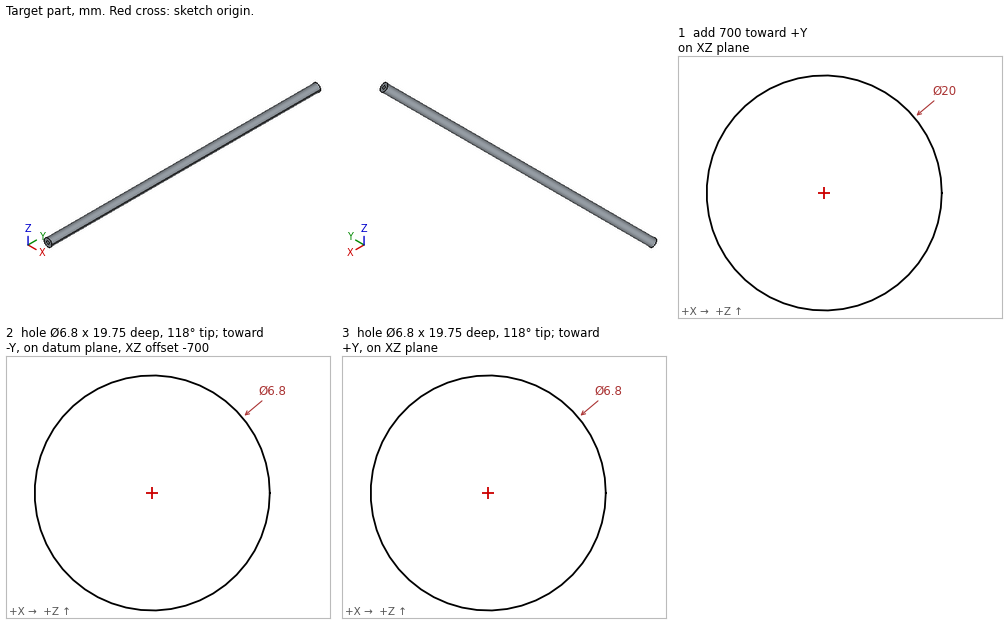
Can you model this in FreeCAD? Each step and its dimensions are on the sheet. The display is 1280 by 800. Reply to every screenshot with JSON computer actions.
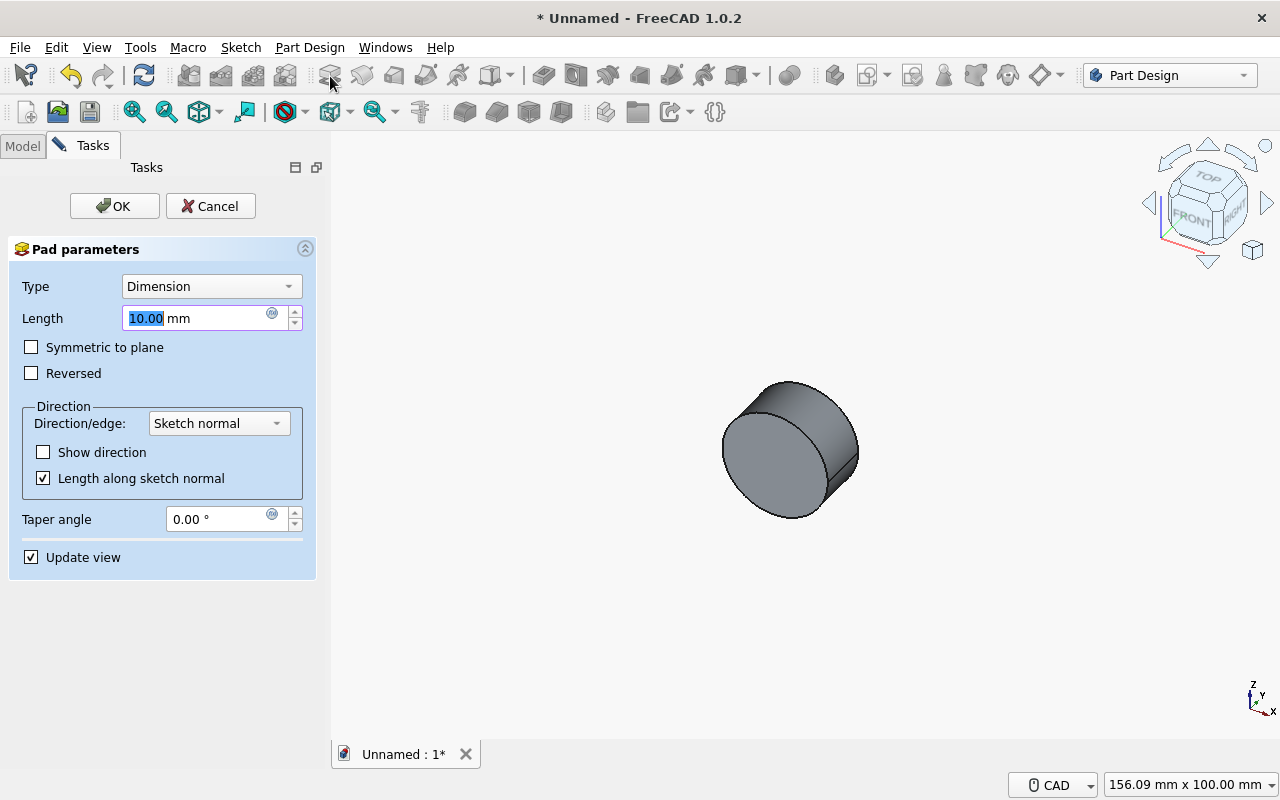
{"action": "type", "text": "700"}
{"action": "key", "text": "Tab"}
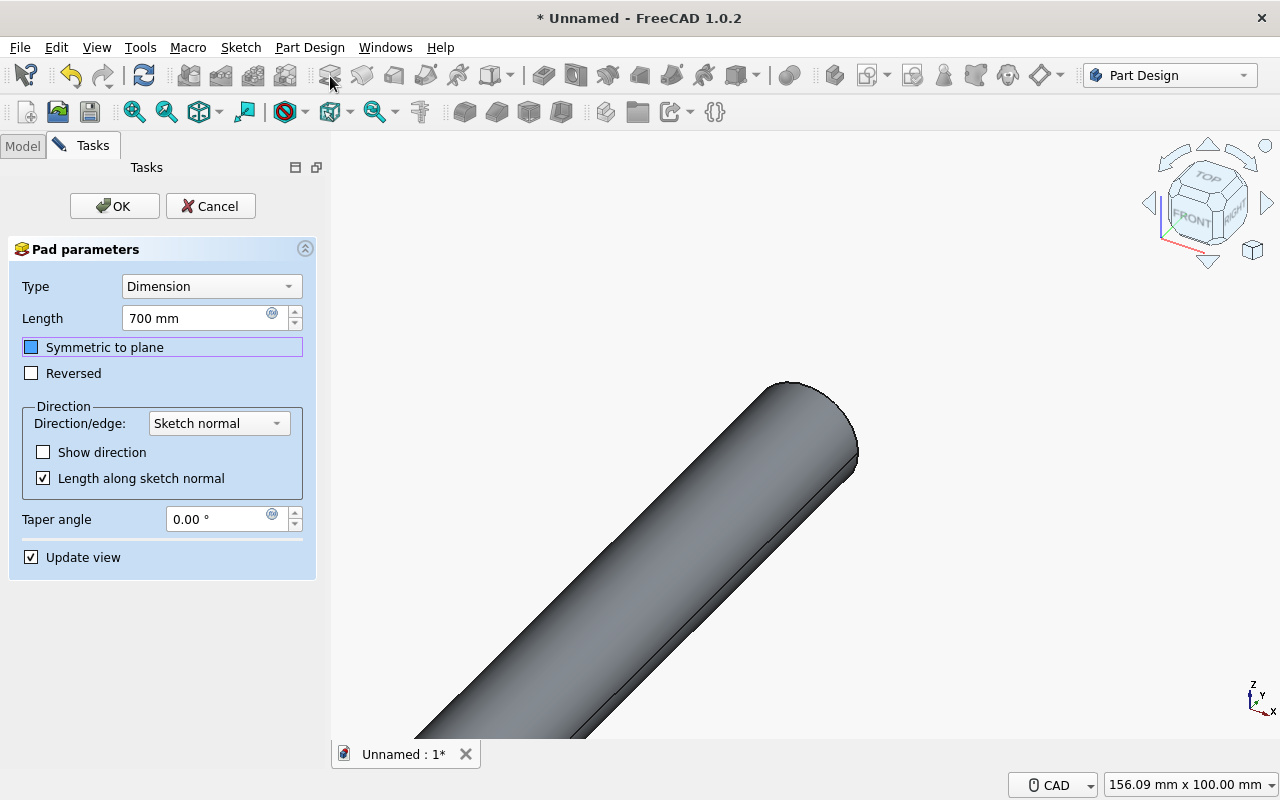
{"action": "left_click", "coordinate": [30, 373]}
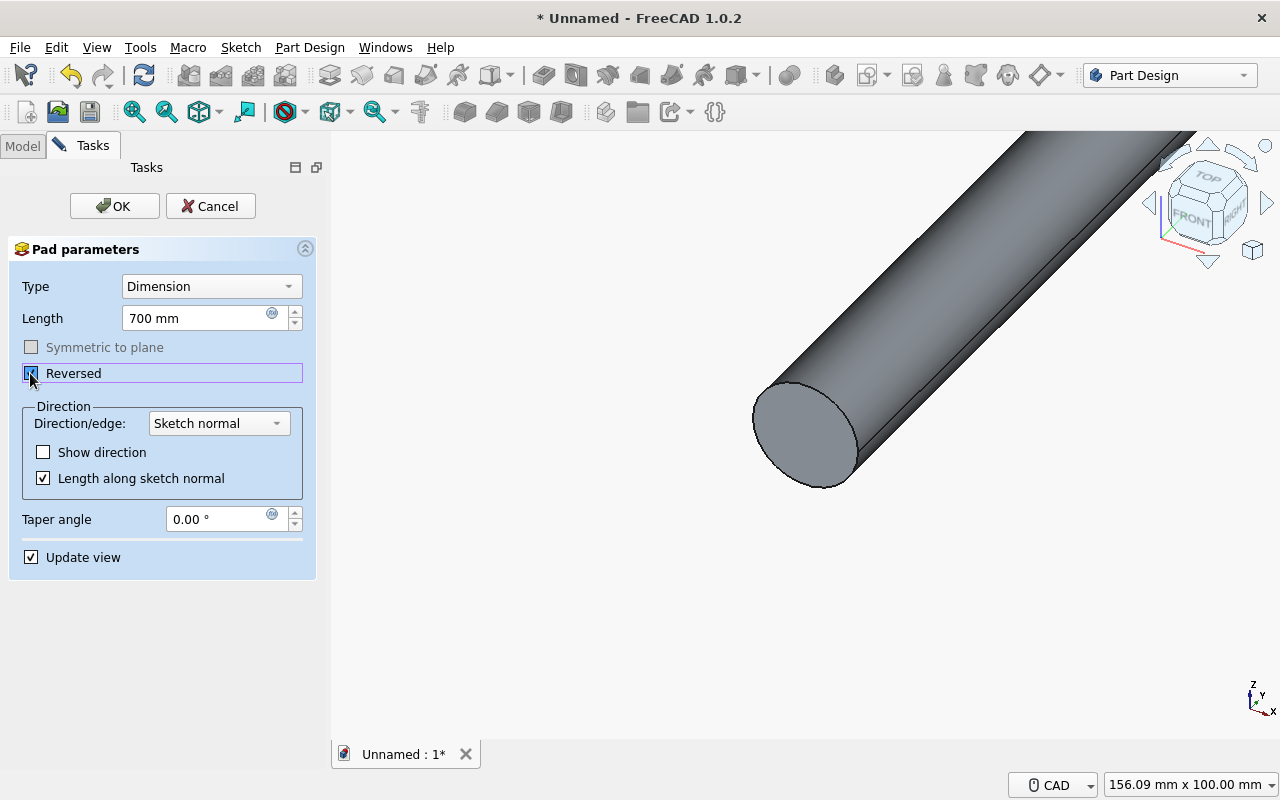
{"action": "left_click", "coordinate": [115, 206]}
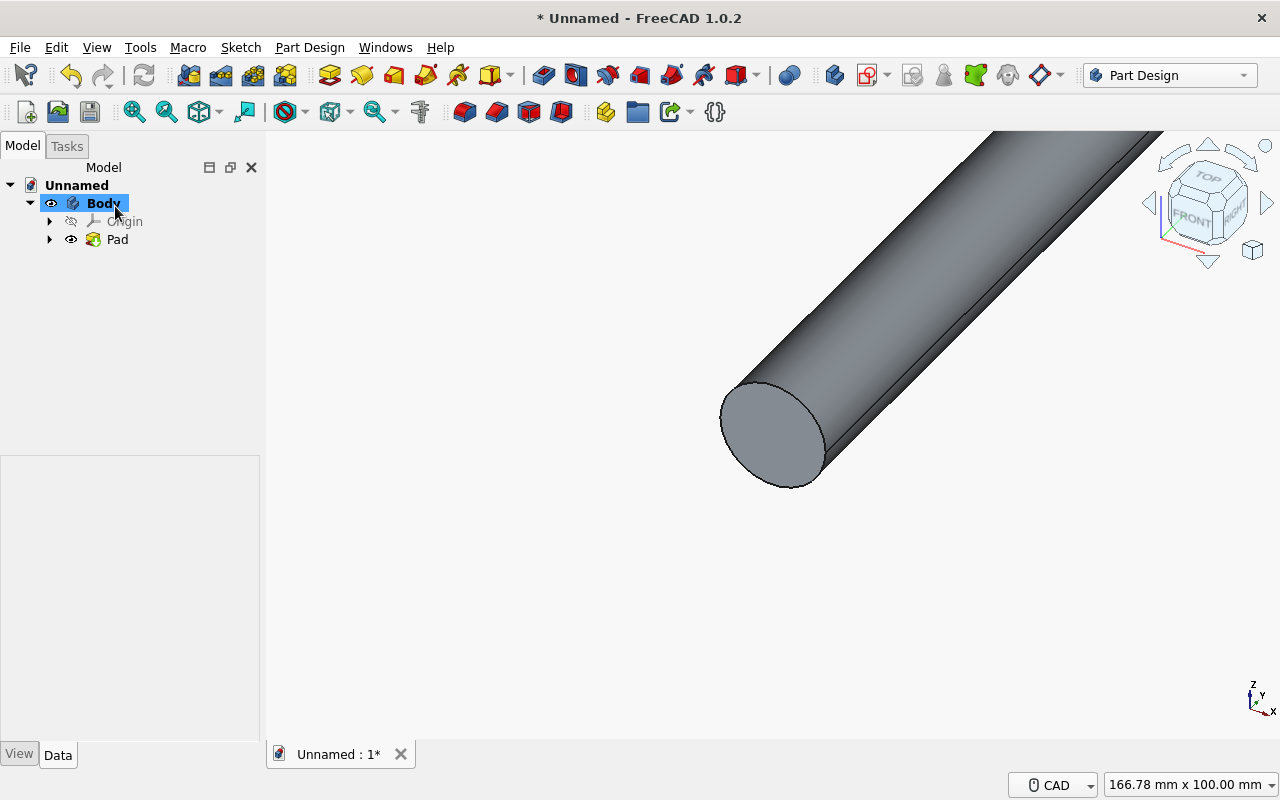
{"action": "left_click", "coordinate": [136, 112]}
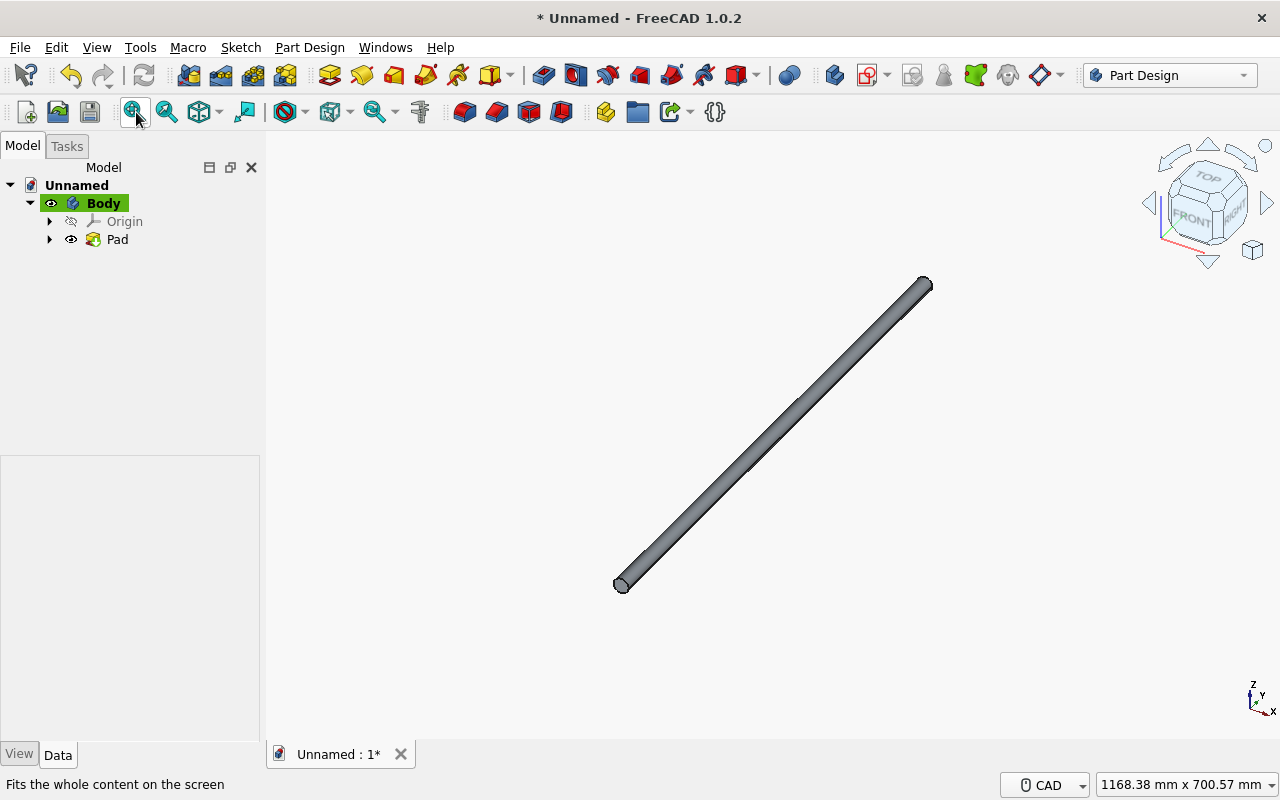
{"action": "key", "text": "4"}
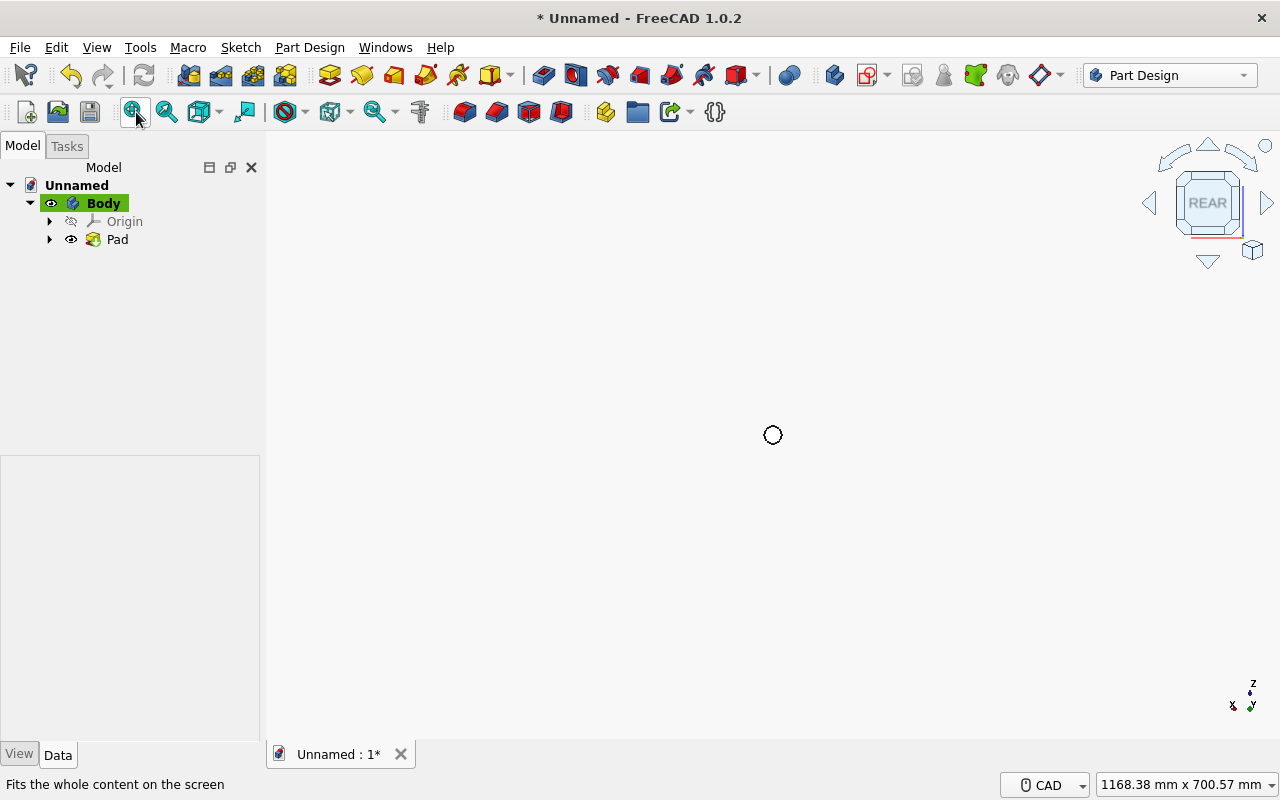
{"action": "left_click", "coordinate": [136, 112]}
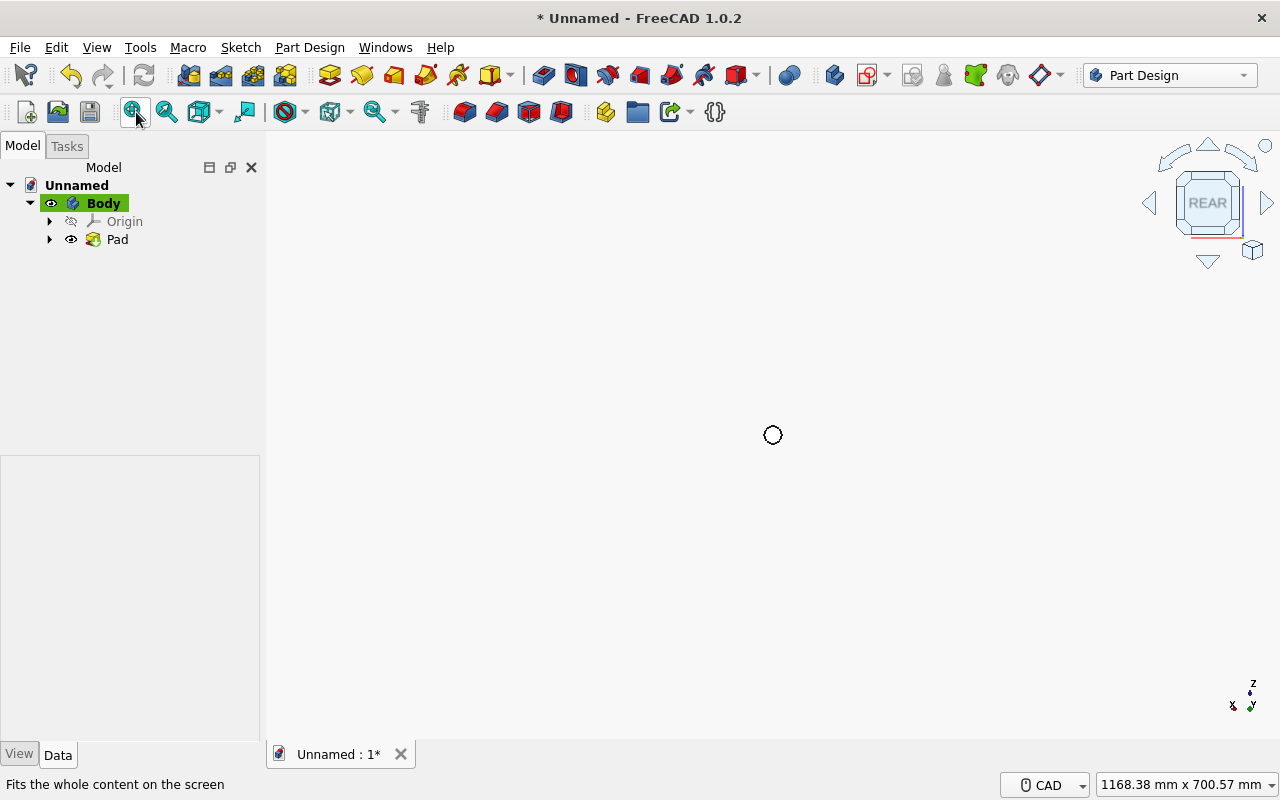
{"action": "key", "text": "5"}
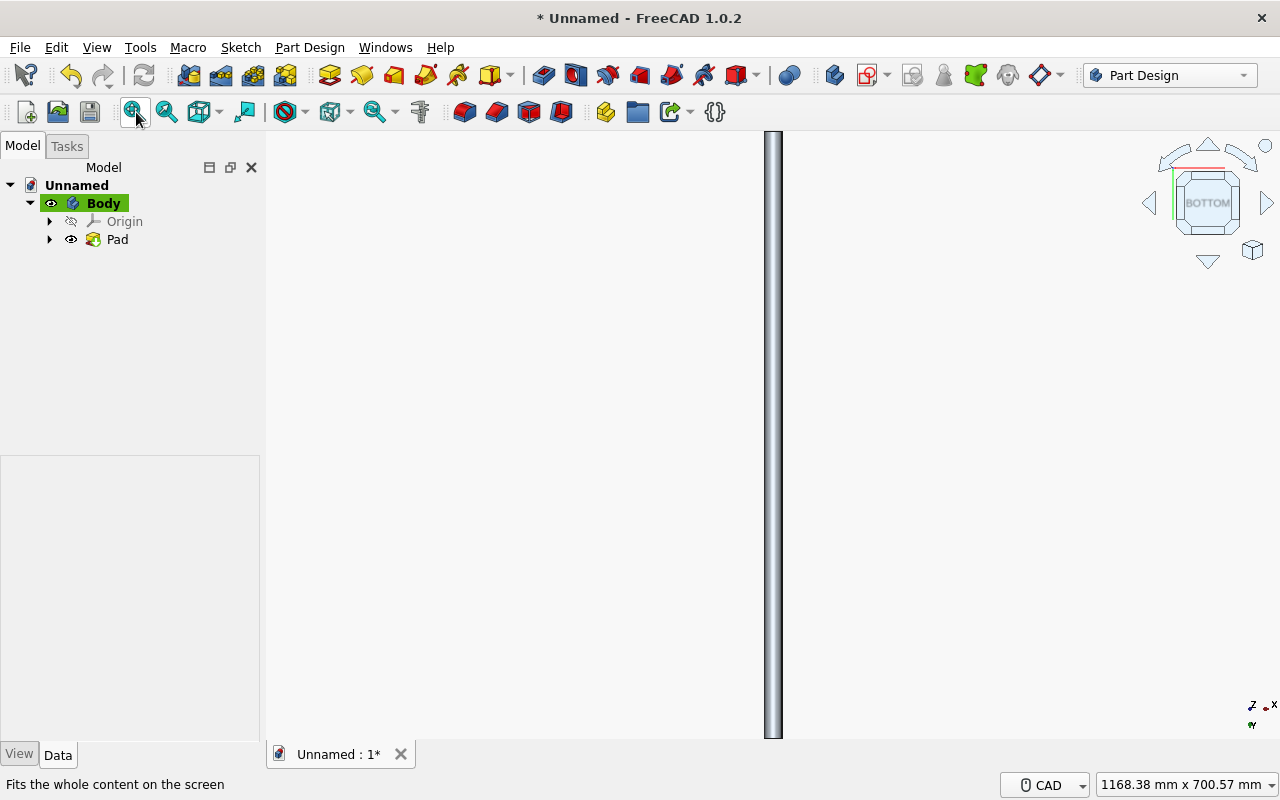
{"action": "left_click", "coordinate": [136, 112]}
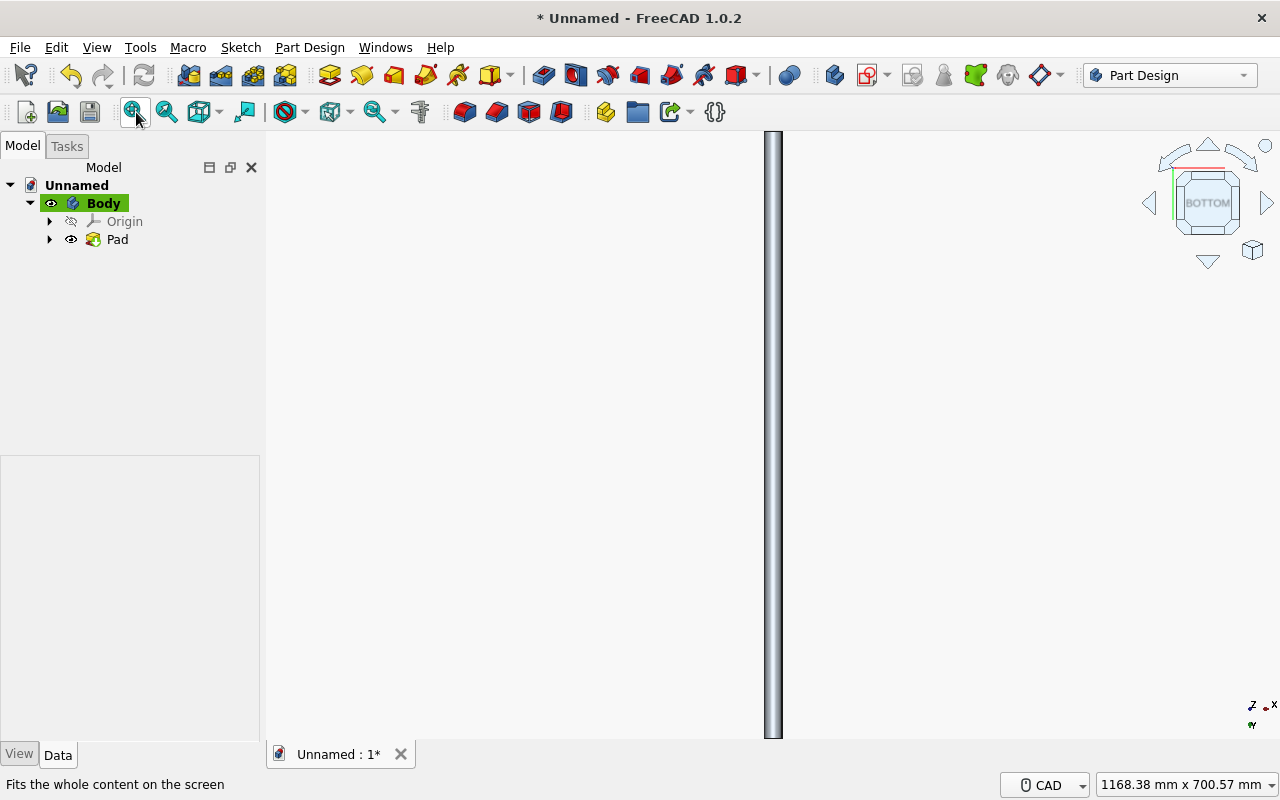
{"action": "key", "text": "3"}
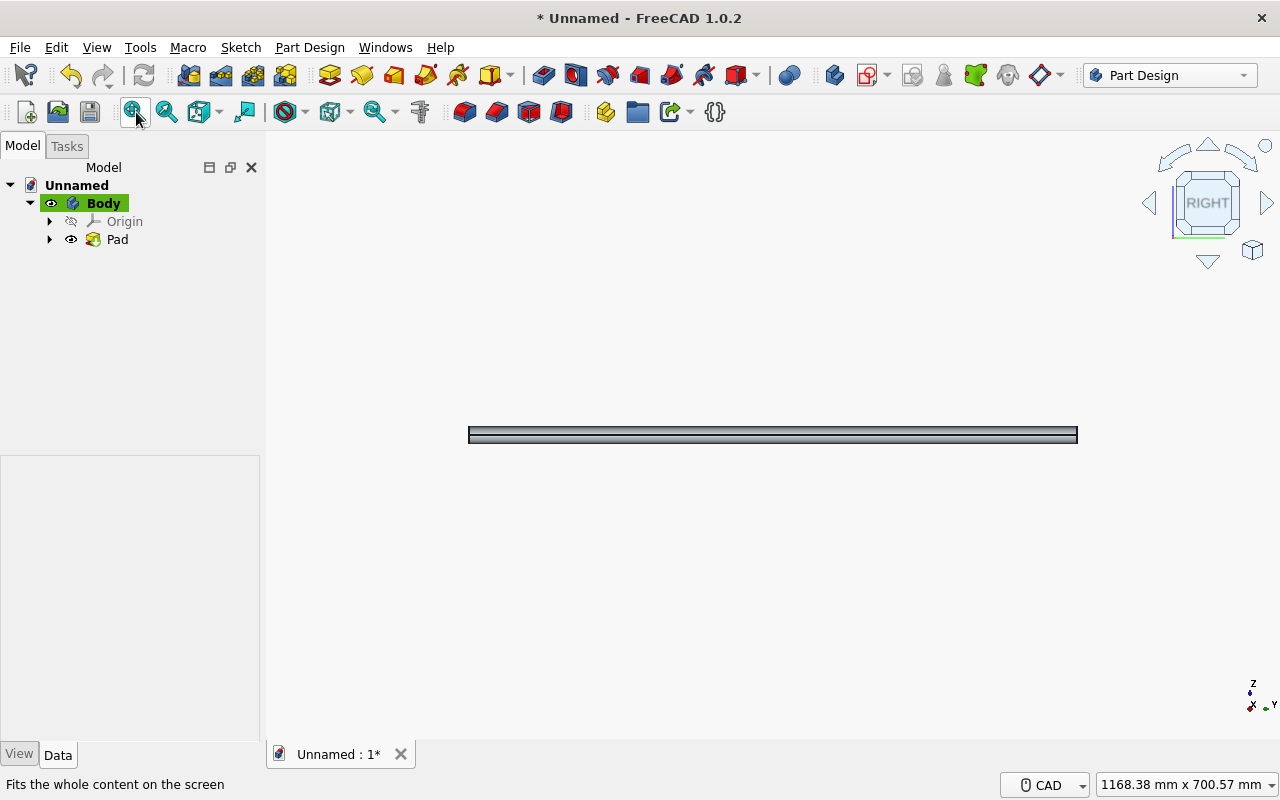
{"action": "left_click", "coordinate": [50, 221]}